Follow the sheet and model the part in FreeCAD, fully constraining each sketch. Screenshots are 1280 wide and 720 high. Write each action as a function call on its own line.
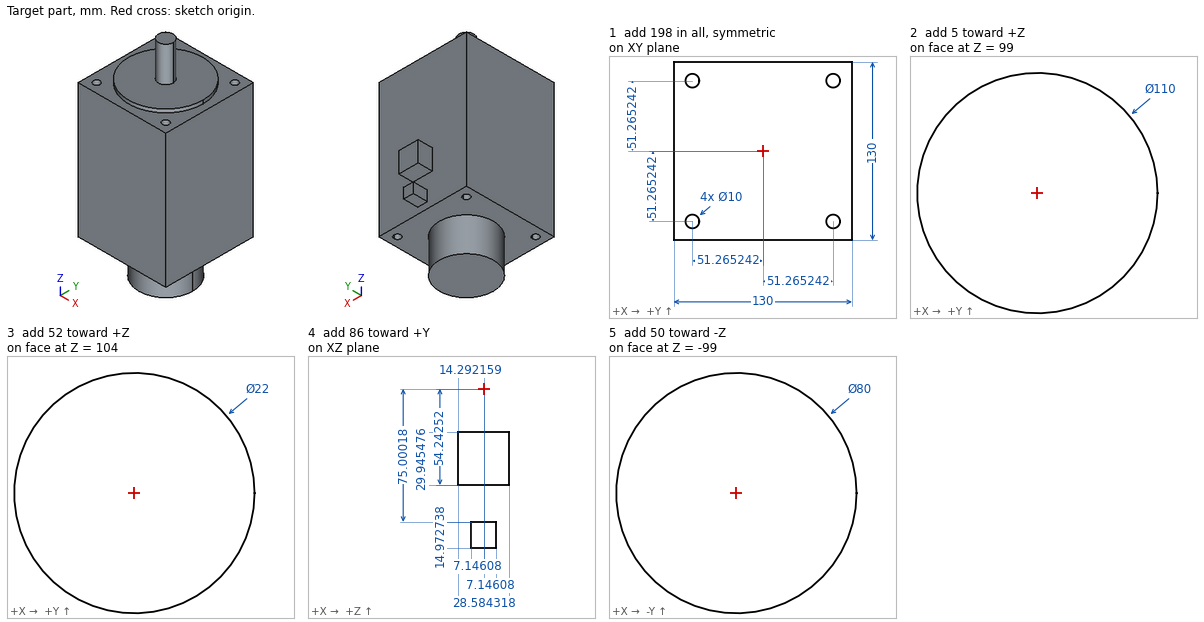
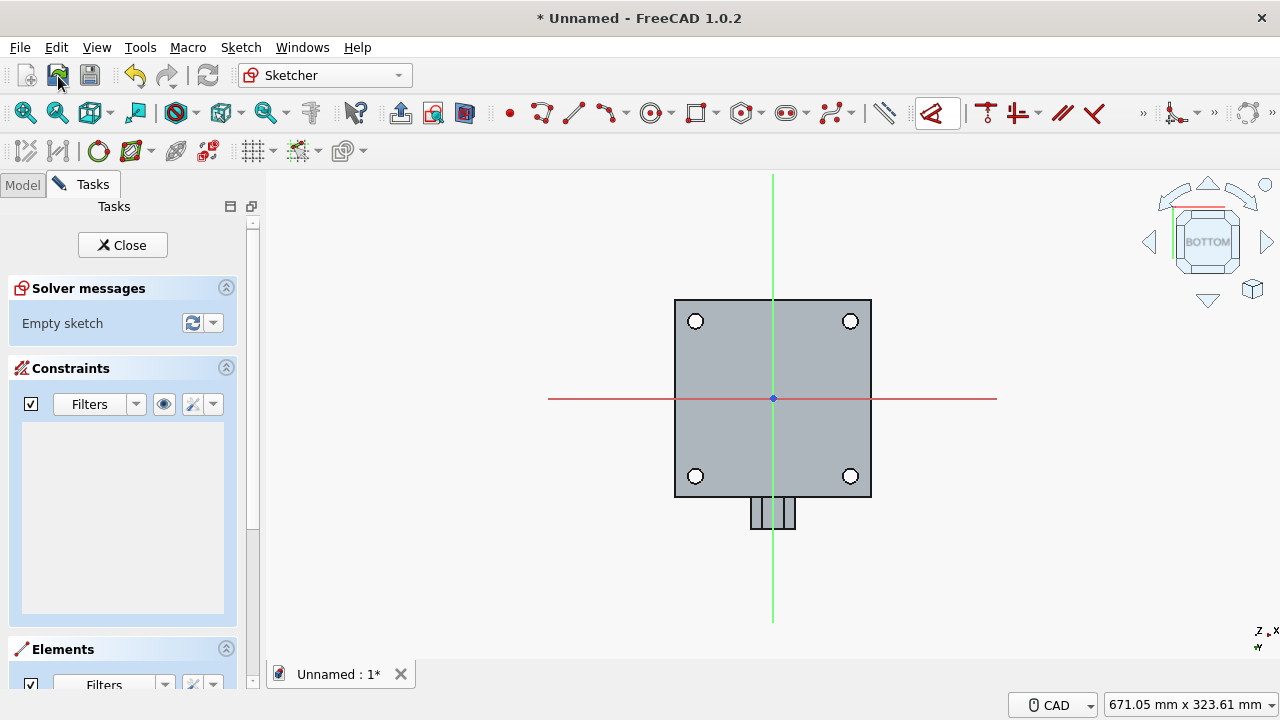
scroll(813, 389, up, 5)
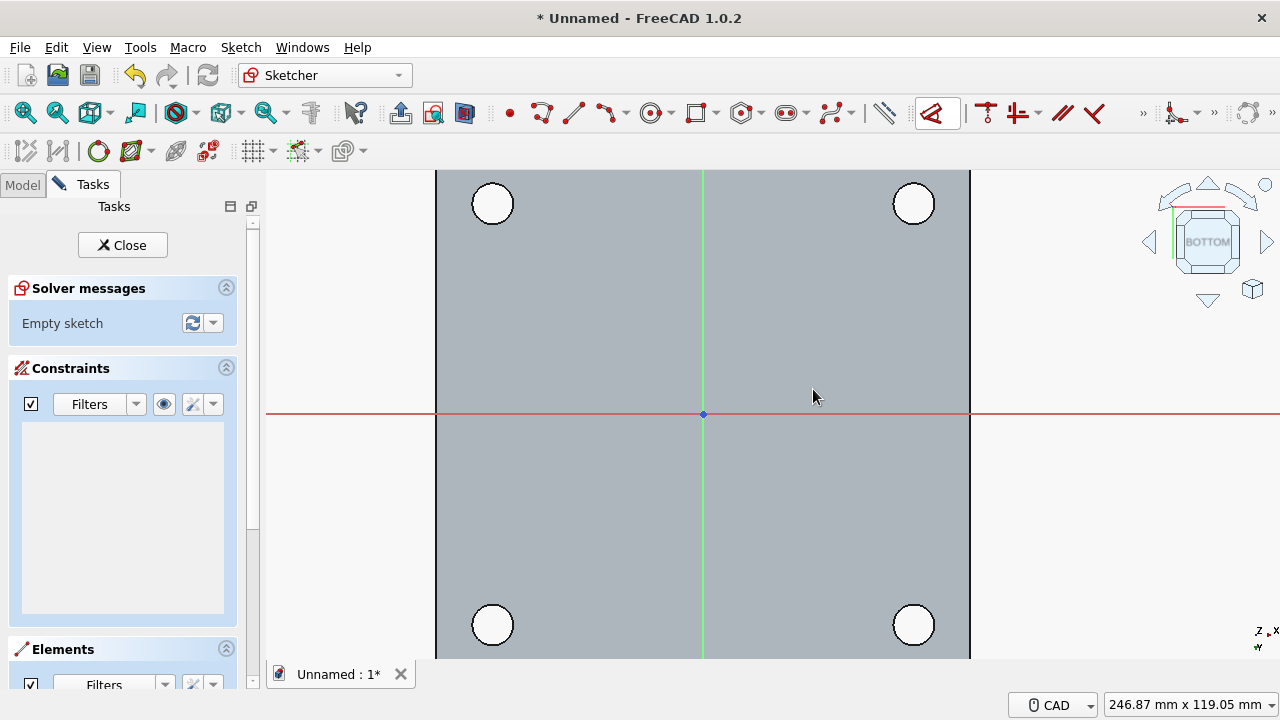
key(g)
key(c)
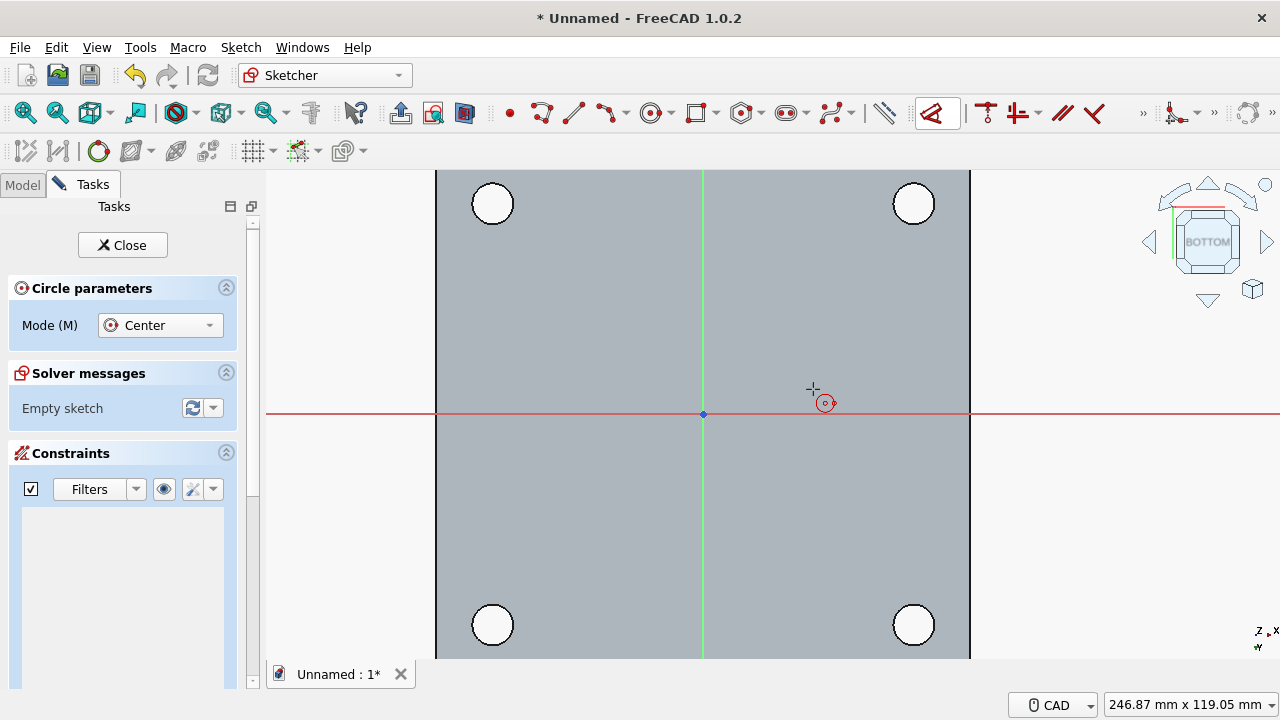
click(703, 414)
click(820, 298)
key(Escape)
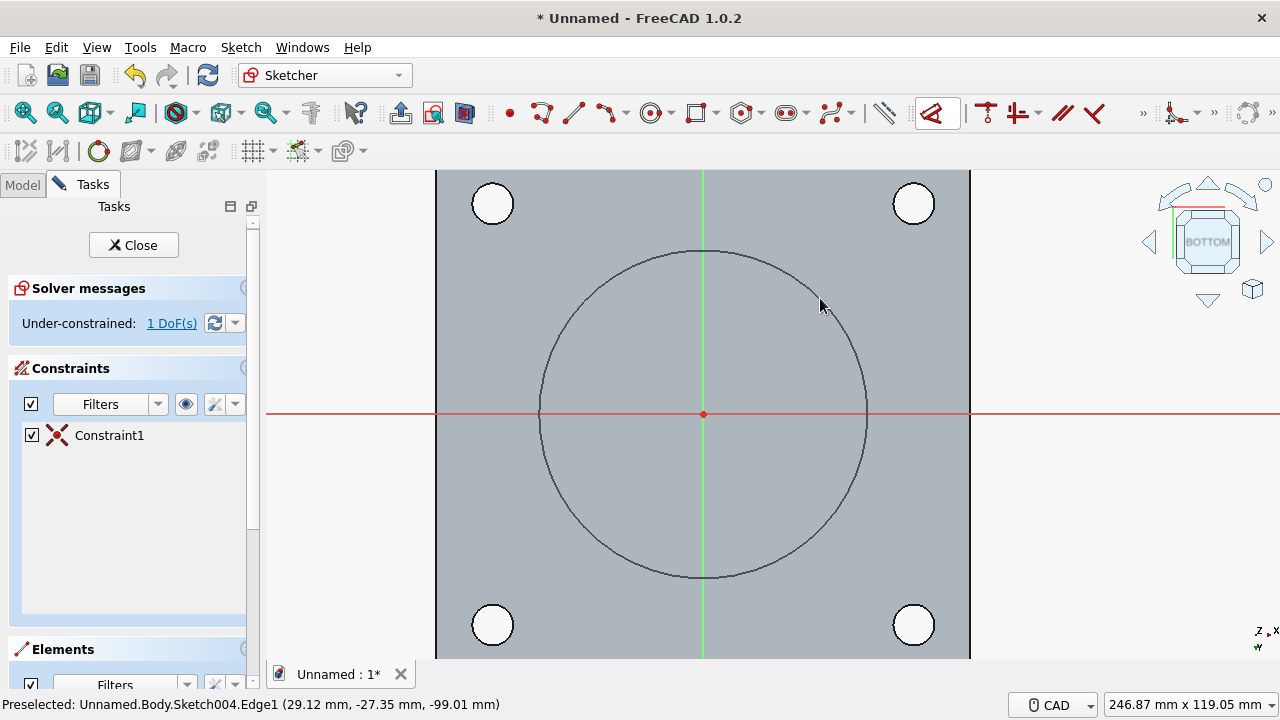
click(819, 298)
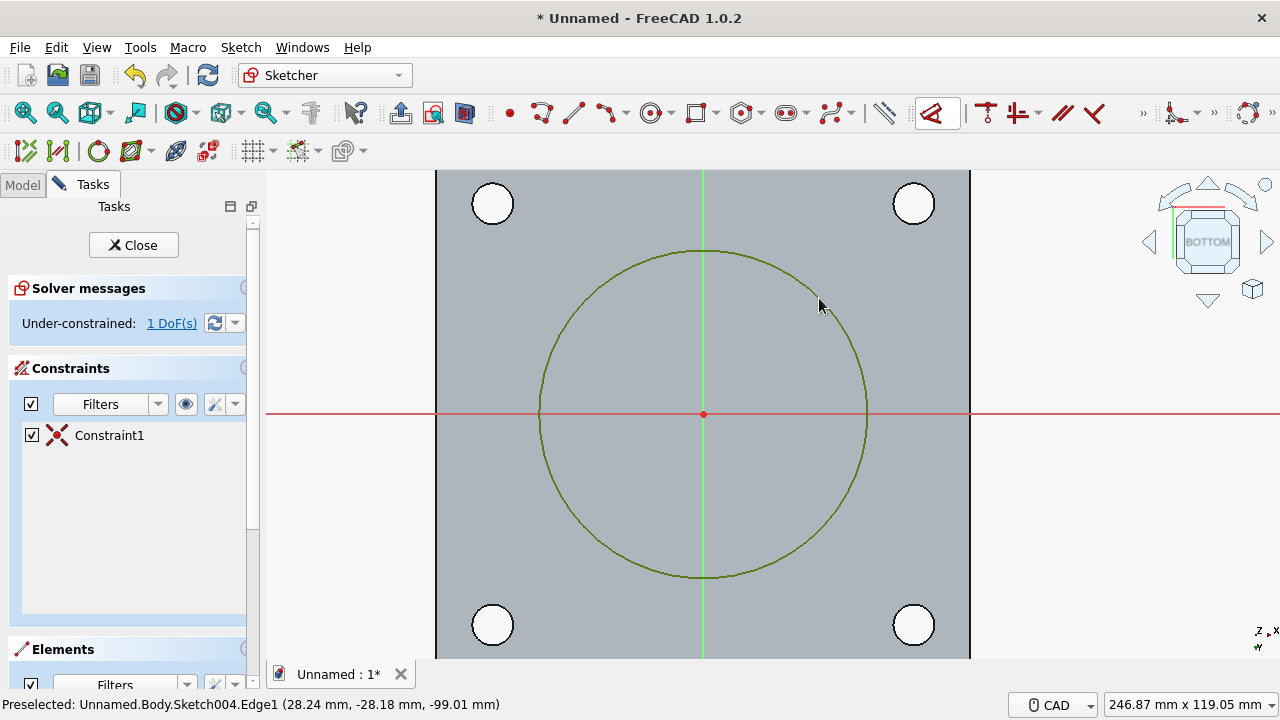
key(k)
key(o)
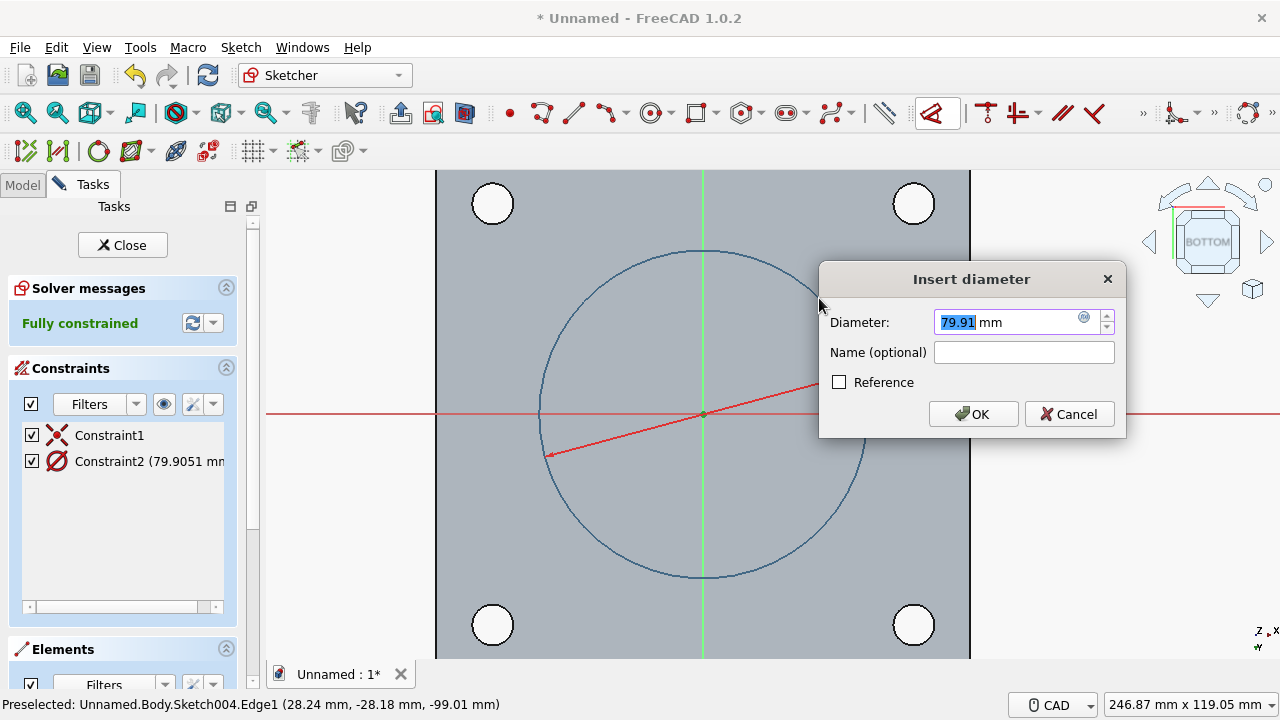
text(80)
key(Return)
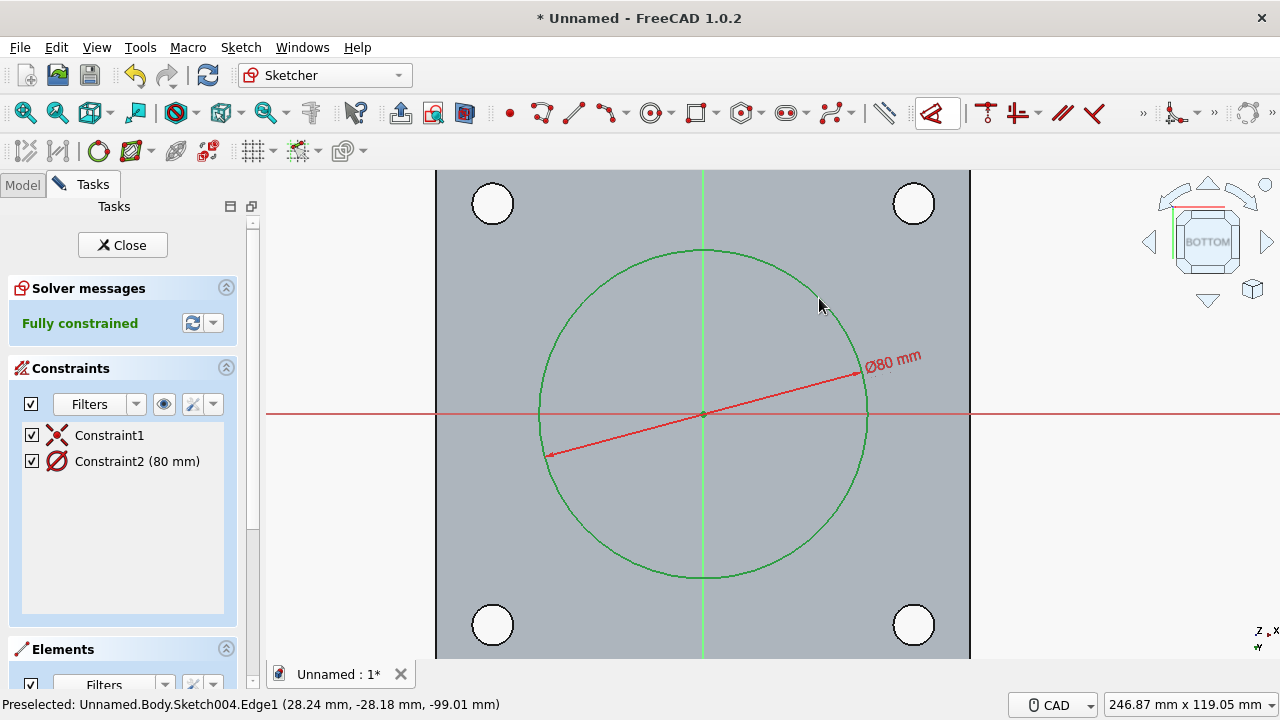
click(123, 245)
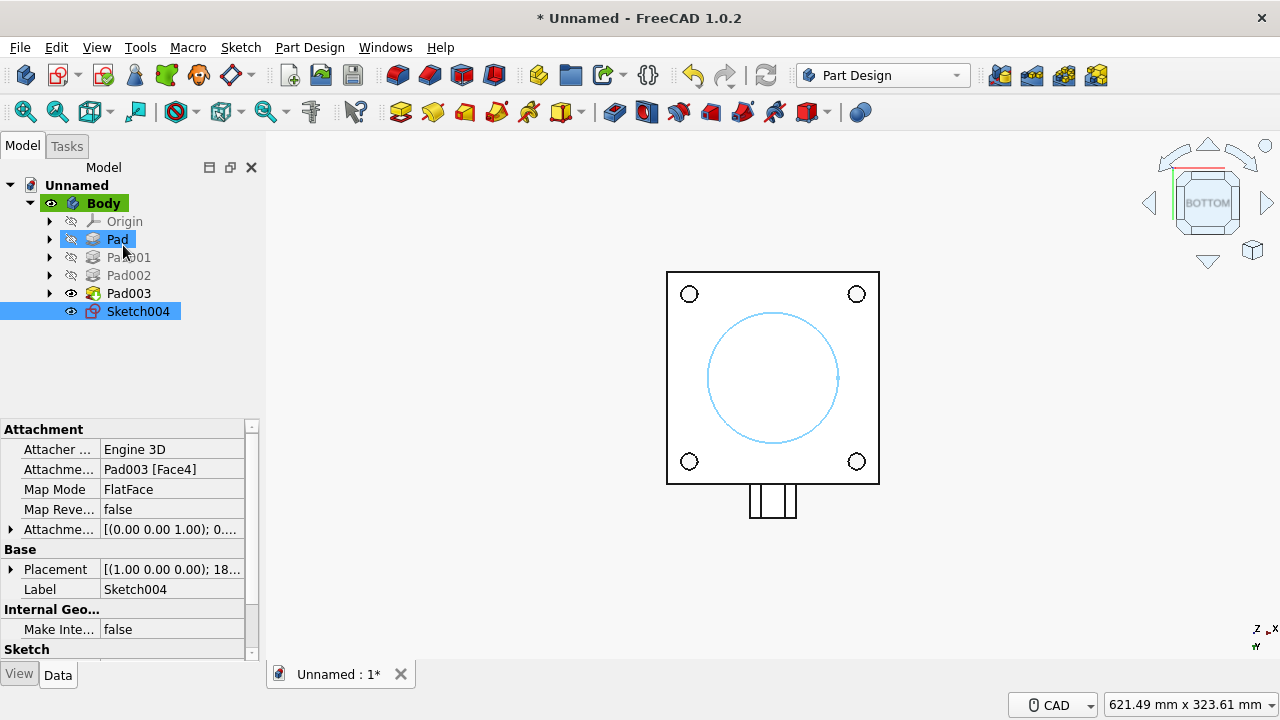
click(402, 112)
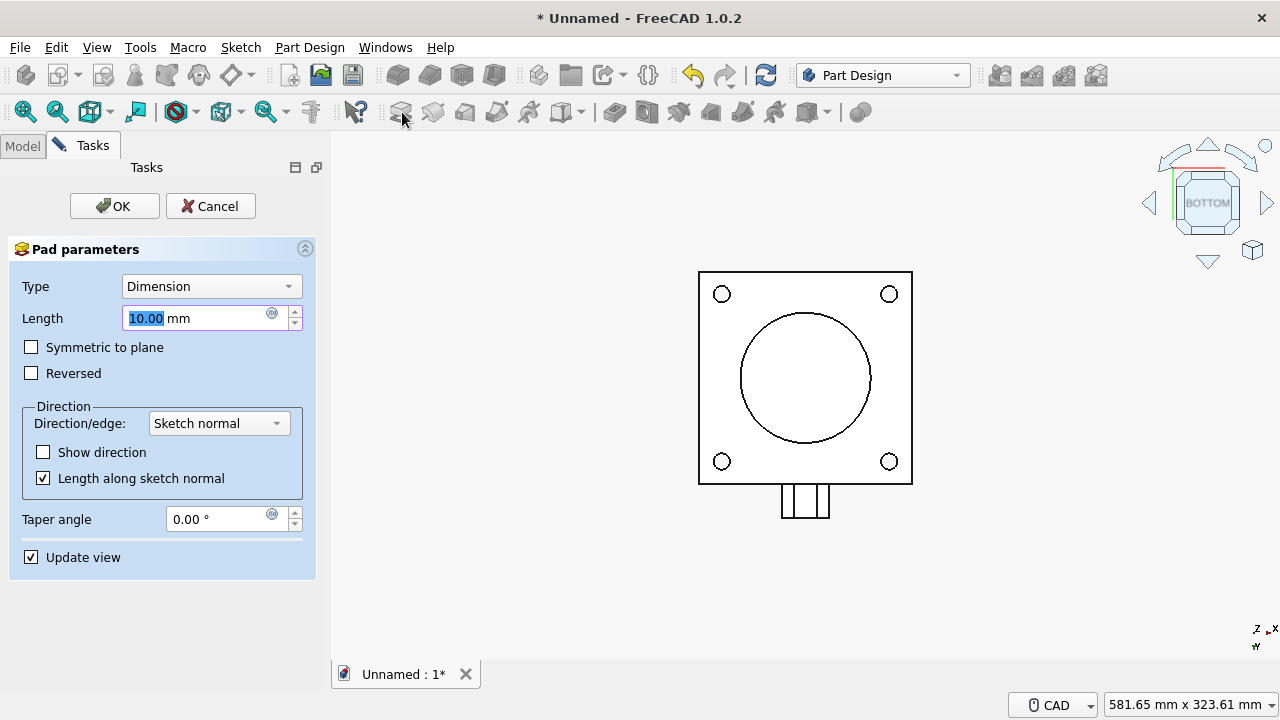
text(50)
key(Tab)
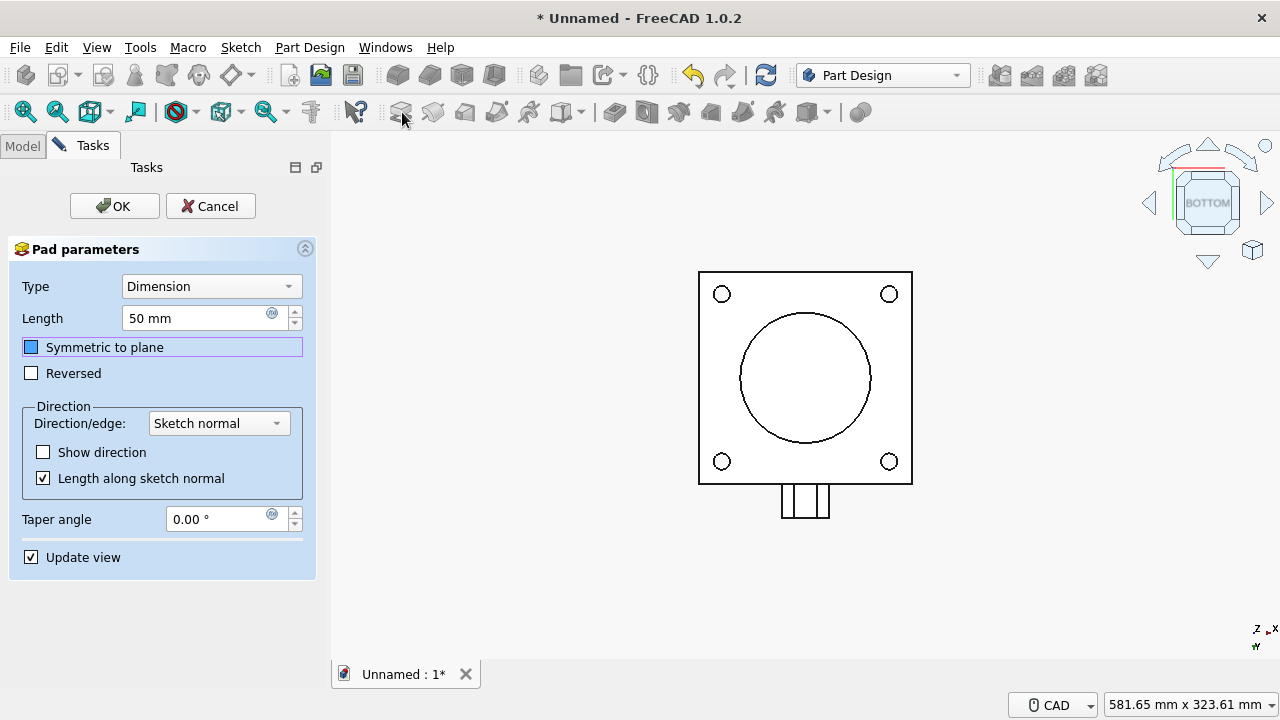
click(115, 206)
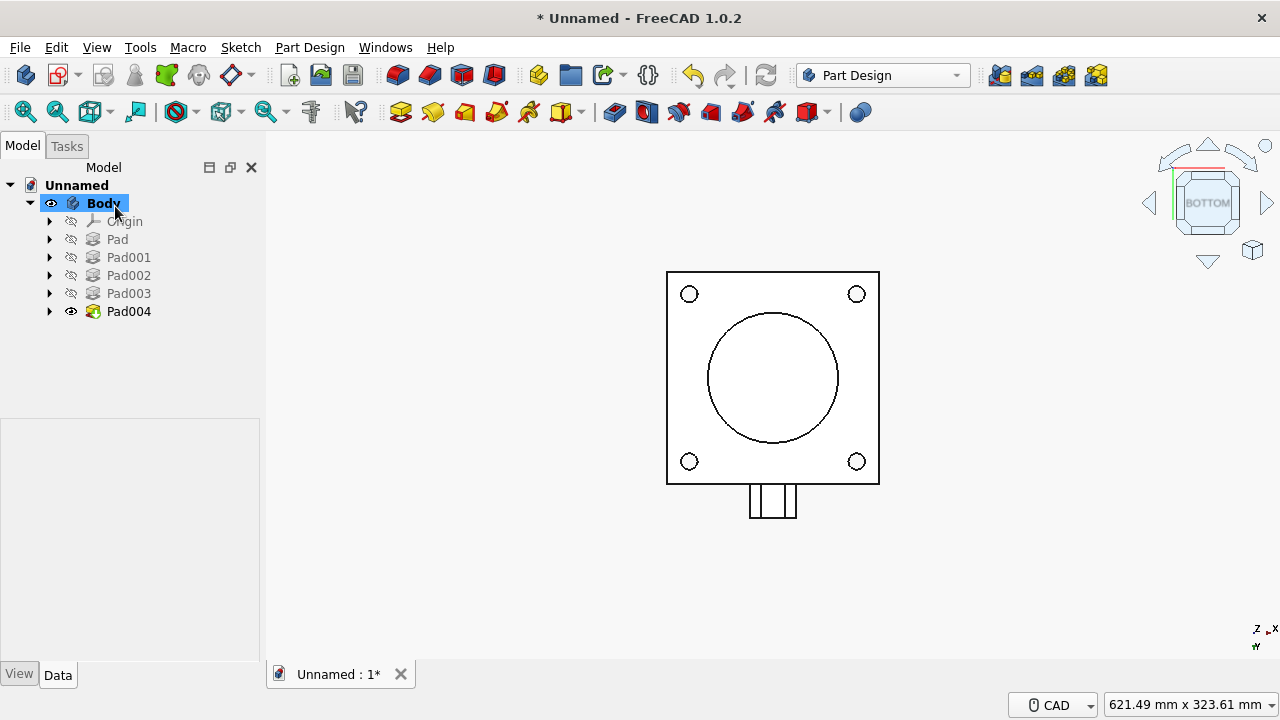
key(0)